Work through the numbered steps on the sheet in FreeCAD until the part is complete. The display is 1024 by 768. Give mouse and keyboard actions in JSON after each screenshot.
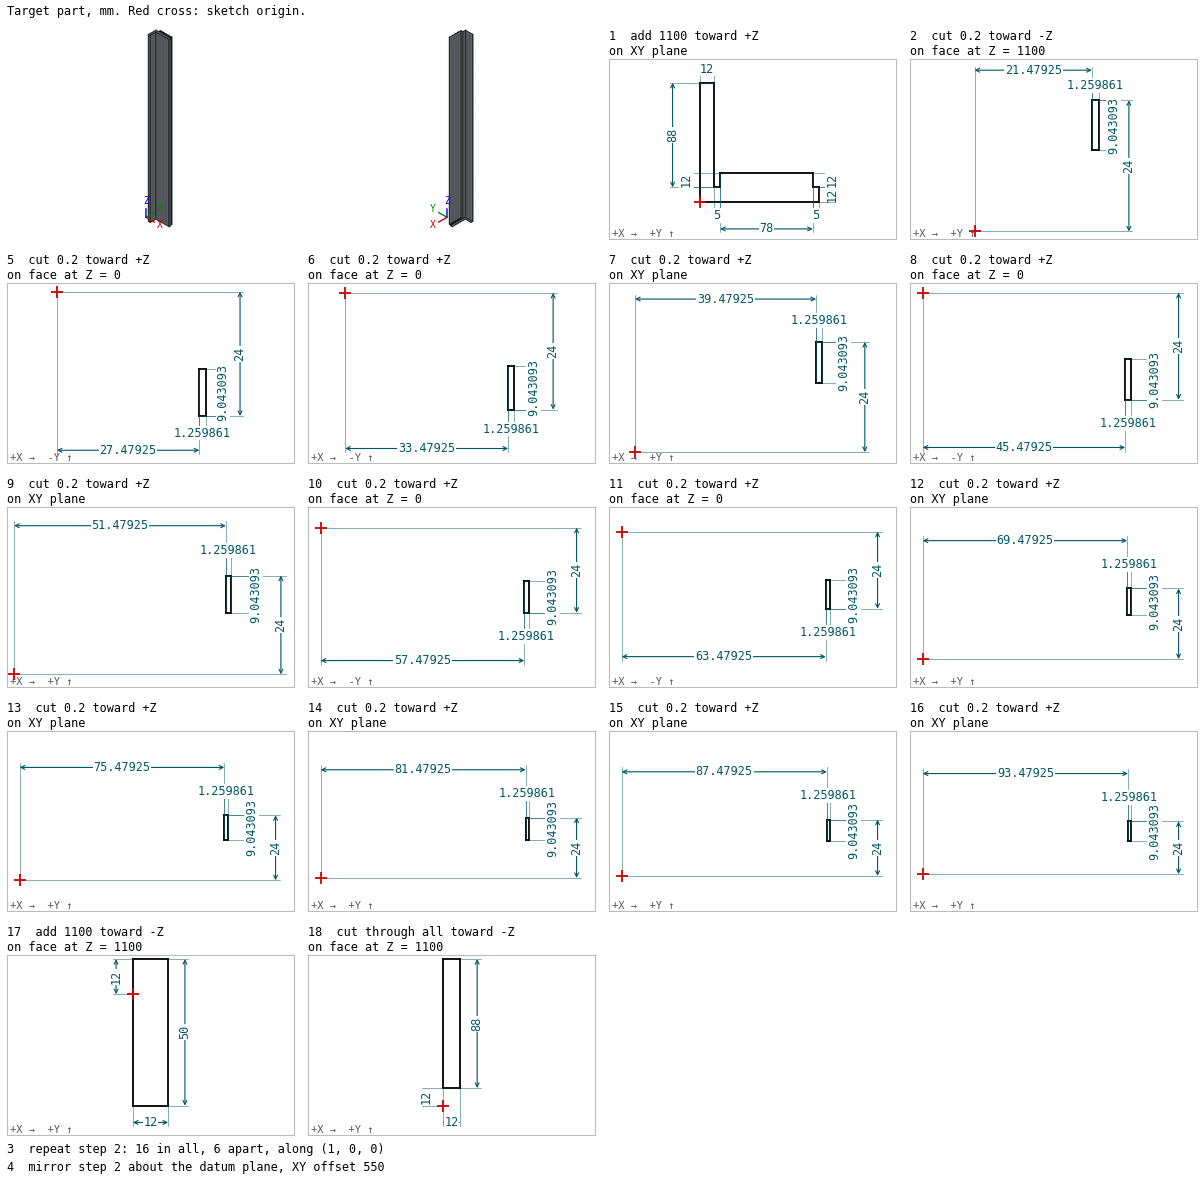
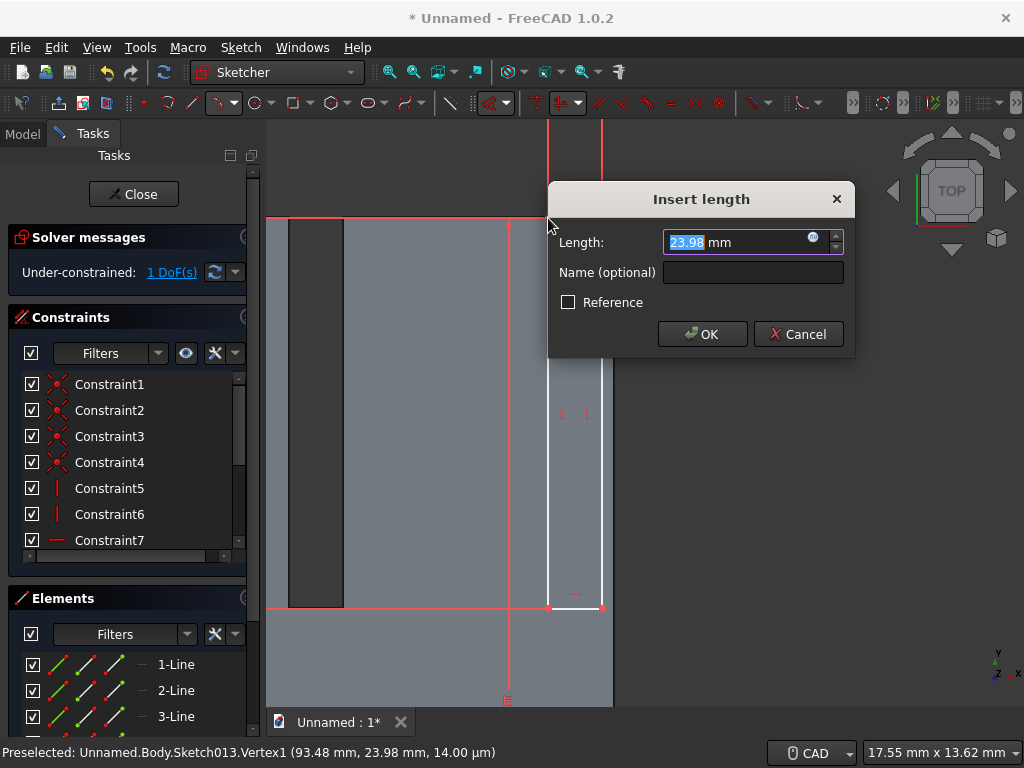
{"action": "type", "text": "24"}
{"action": "key", "text": "Return"}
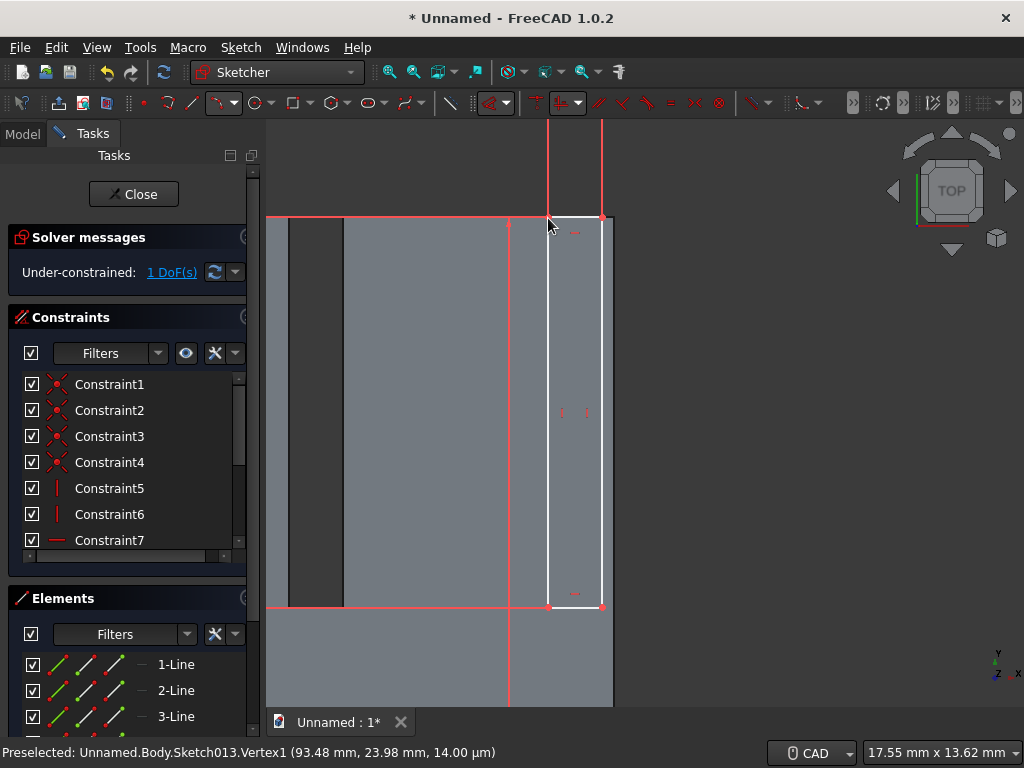
{"action": "left_click", "coordinate": [548, 217]}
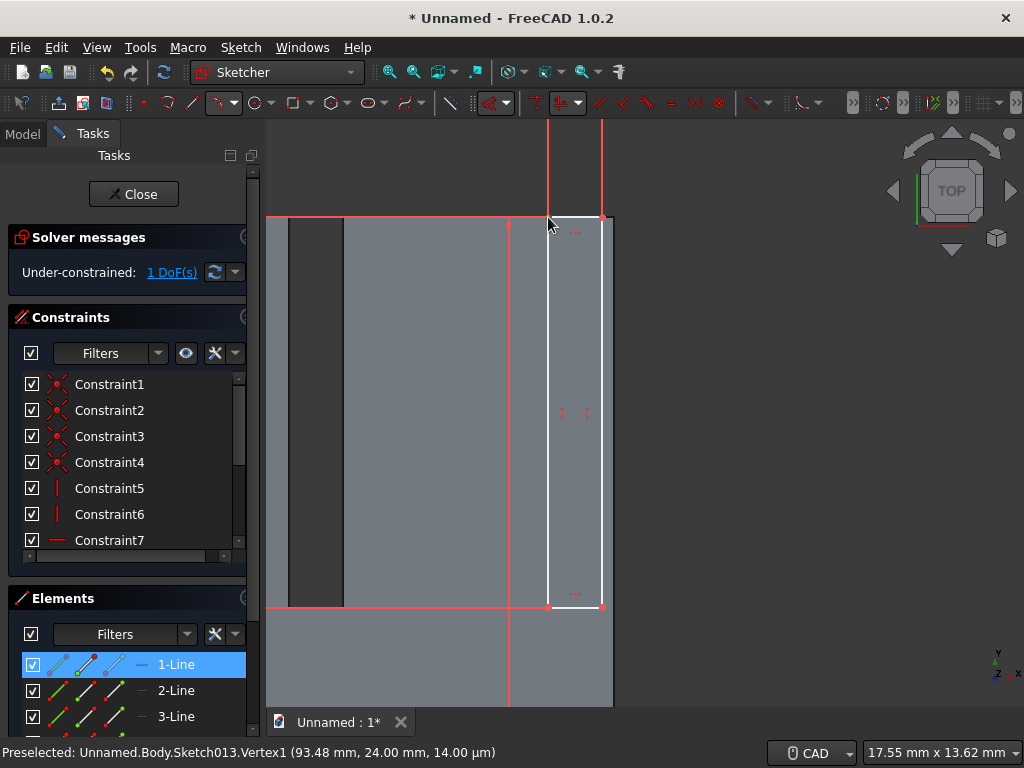
{"action": "key", "text": "l"}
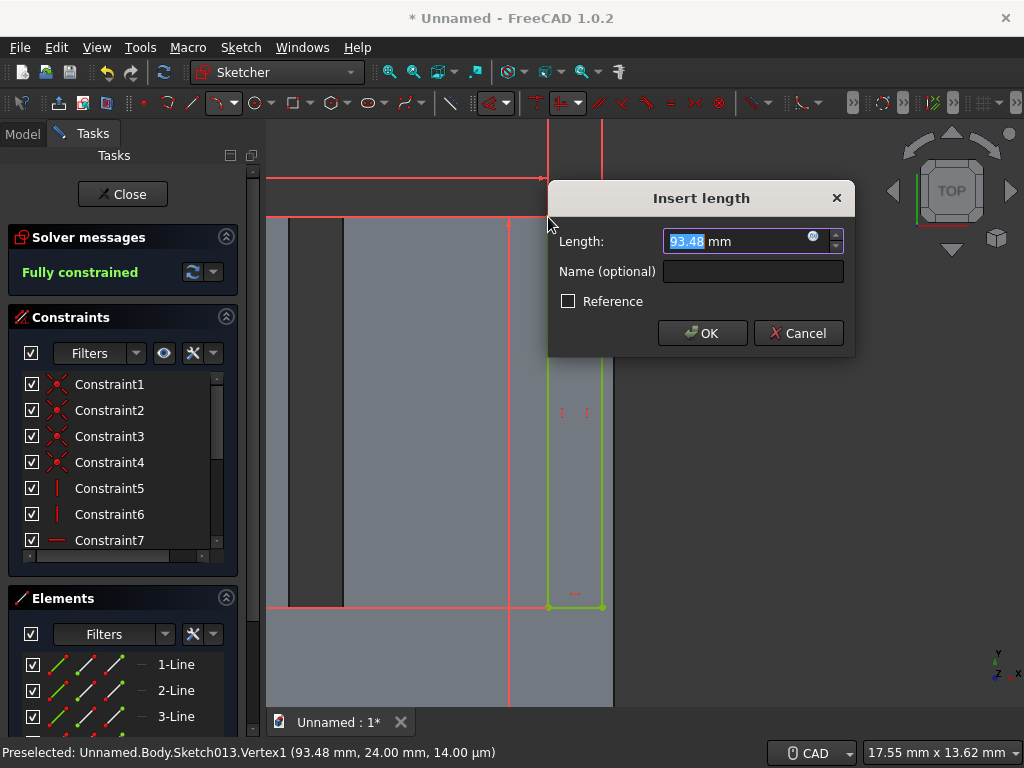
{"action": "type", "text": "93.47925"}
{"action": "key", "text": "Return"}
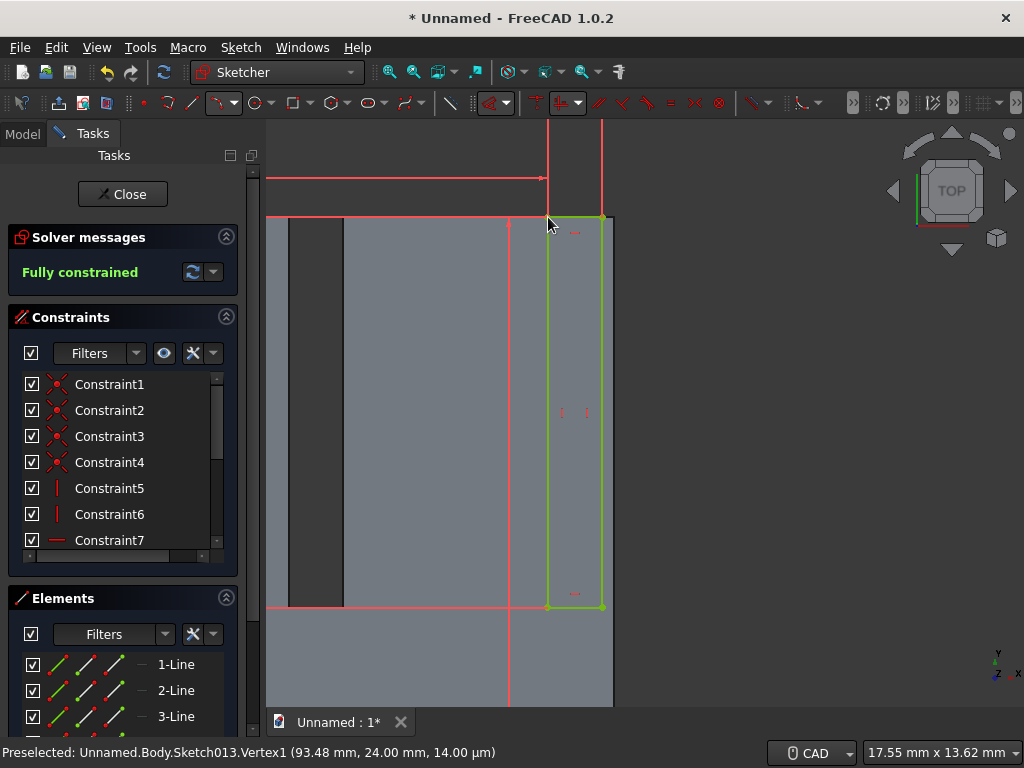
{"action": "left_click", "coordinate": [123, 194]}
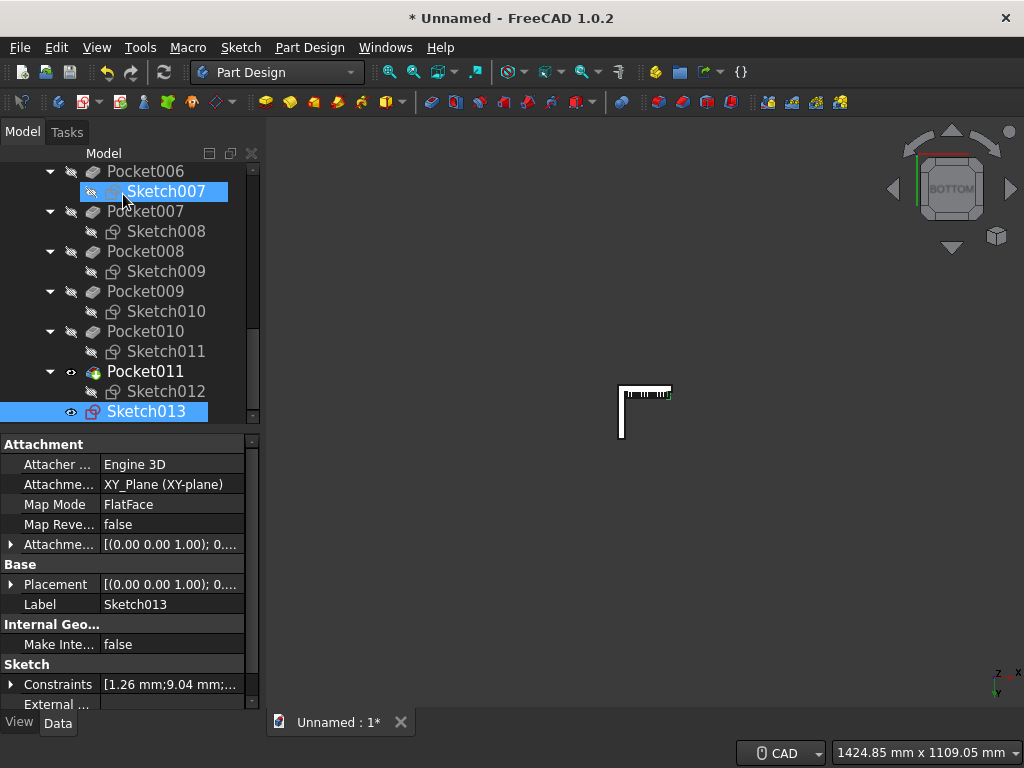
{"action": "left_click", "coordinate": [432, 102]}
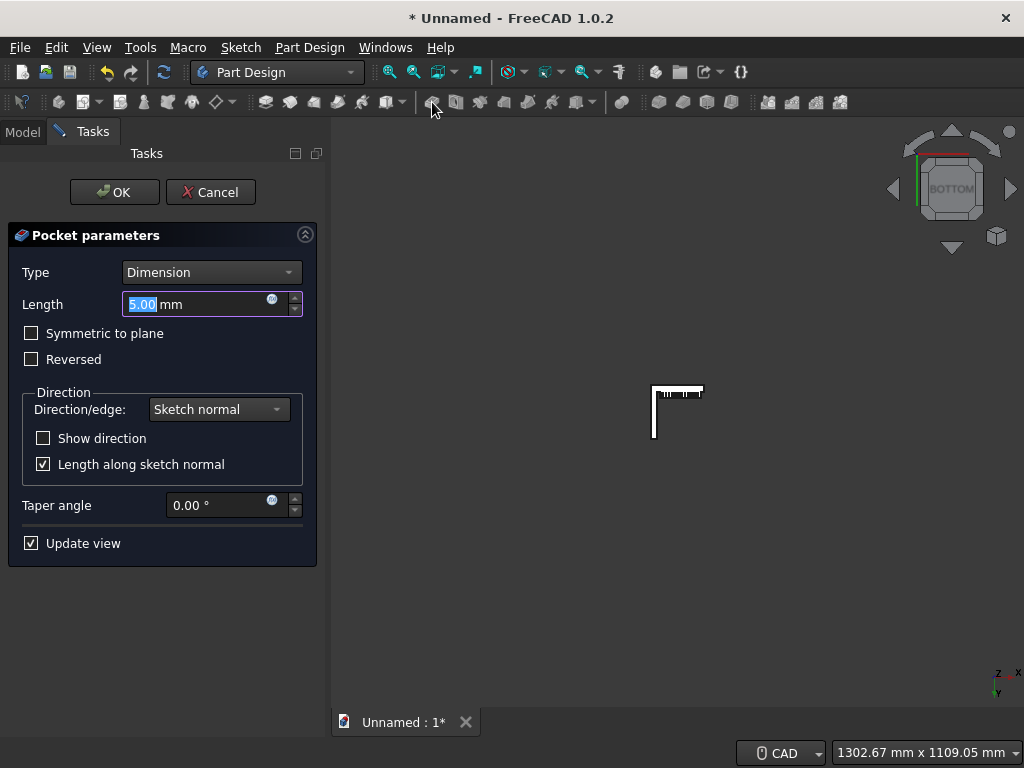
{"action": "type", "text": "0.2"}
{"action": "key", "text": "Tab"}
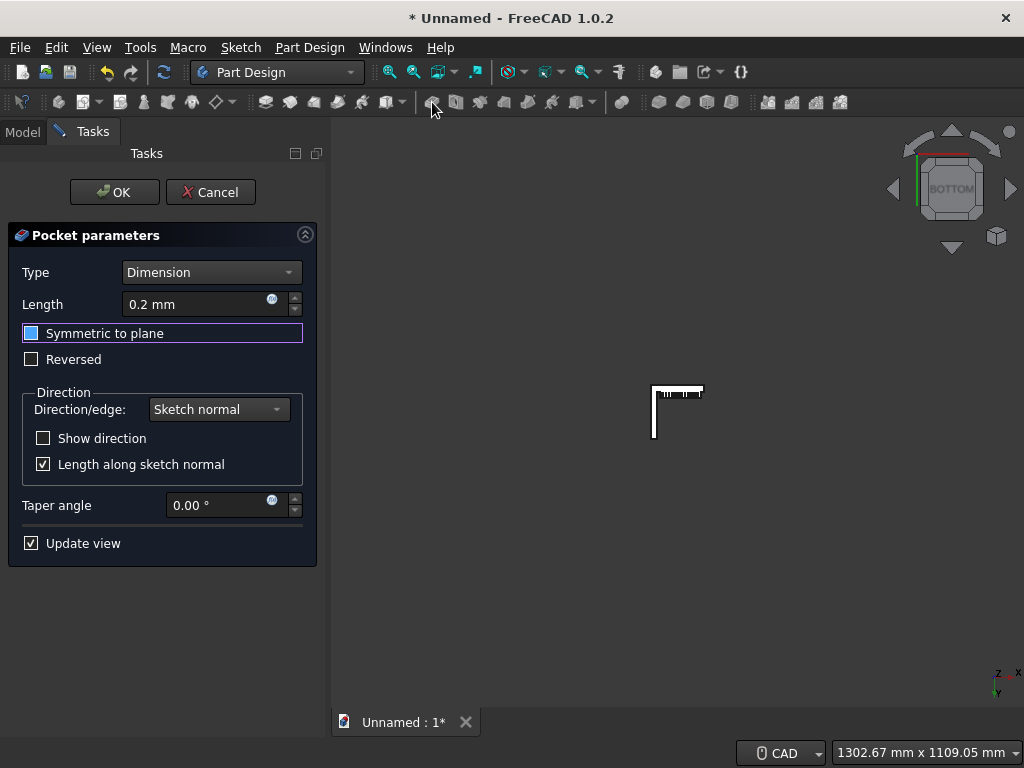
{"action": "left_click", "coordinate": [30, 359]}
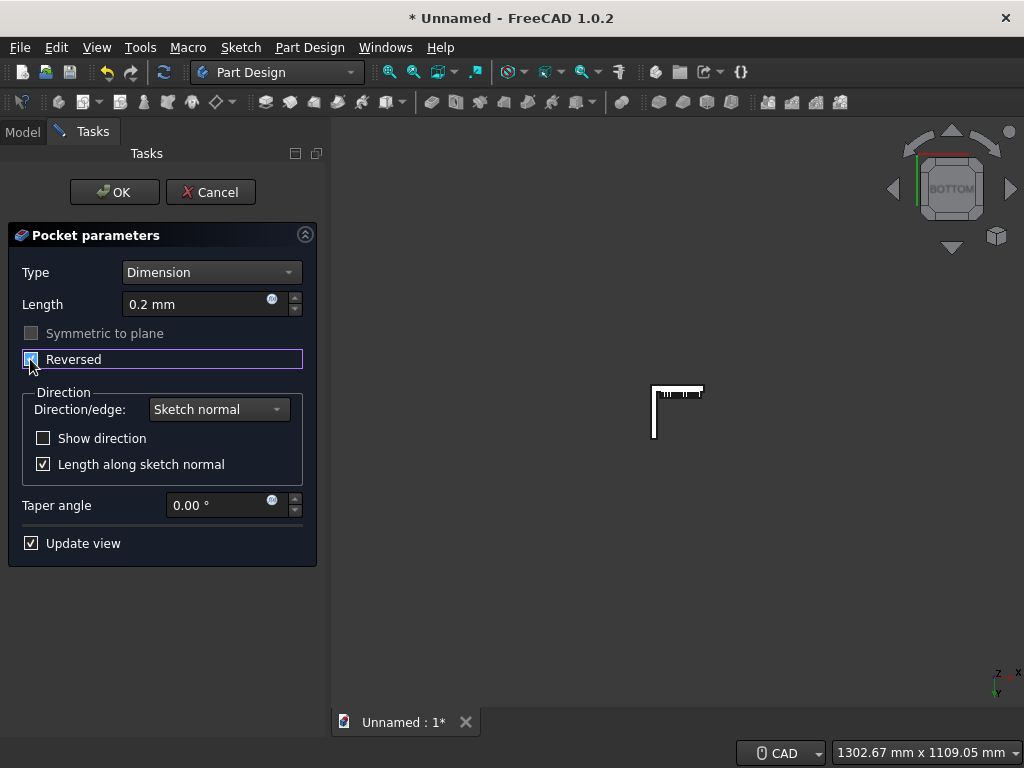
{"action": "left_click", "coordinate": [115, 192]}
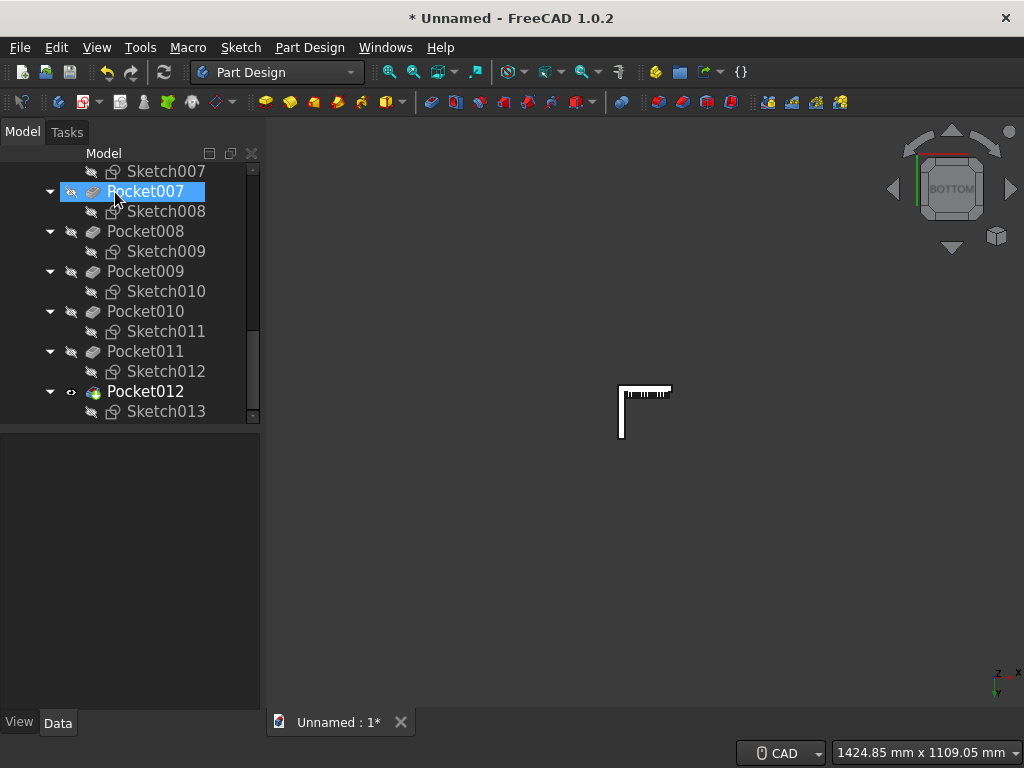
{"action": "left_click", "coordinate": [390, 72]}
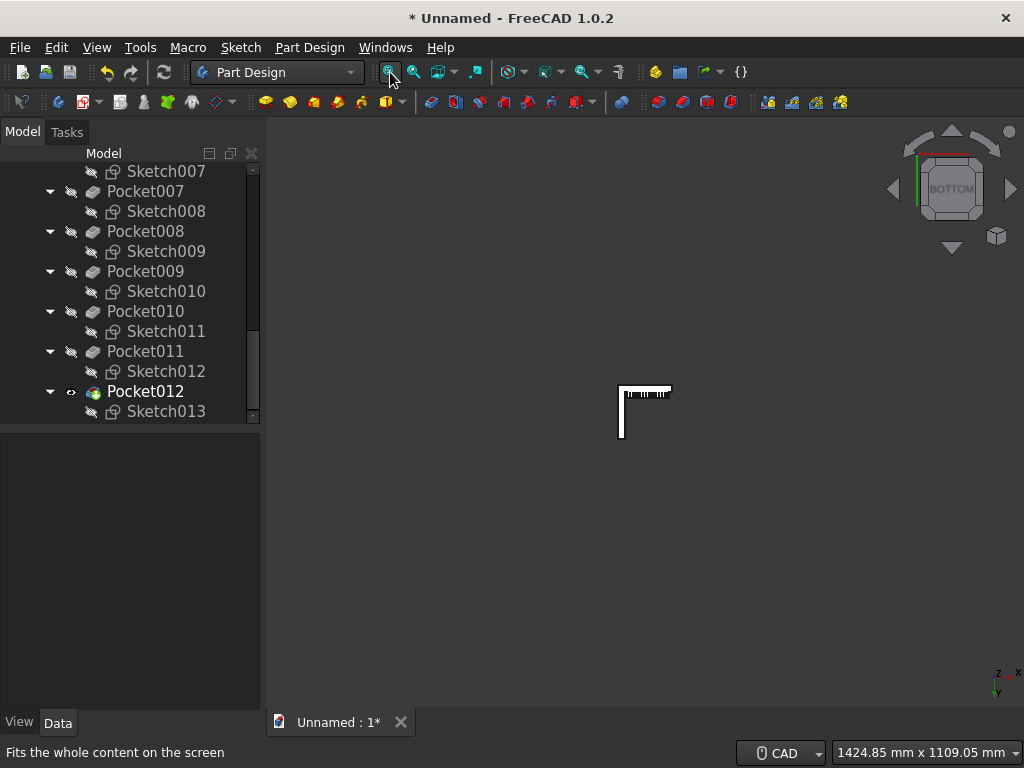
{"action": "key", "text": "0"}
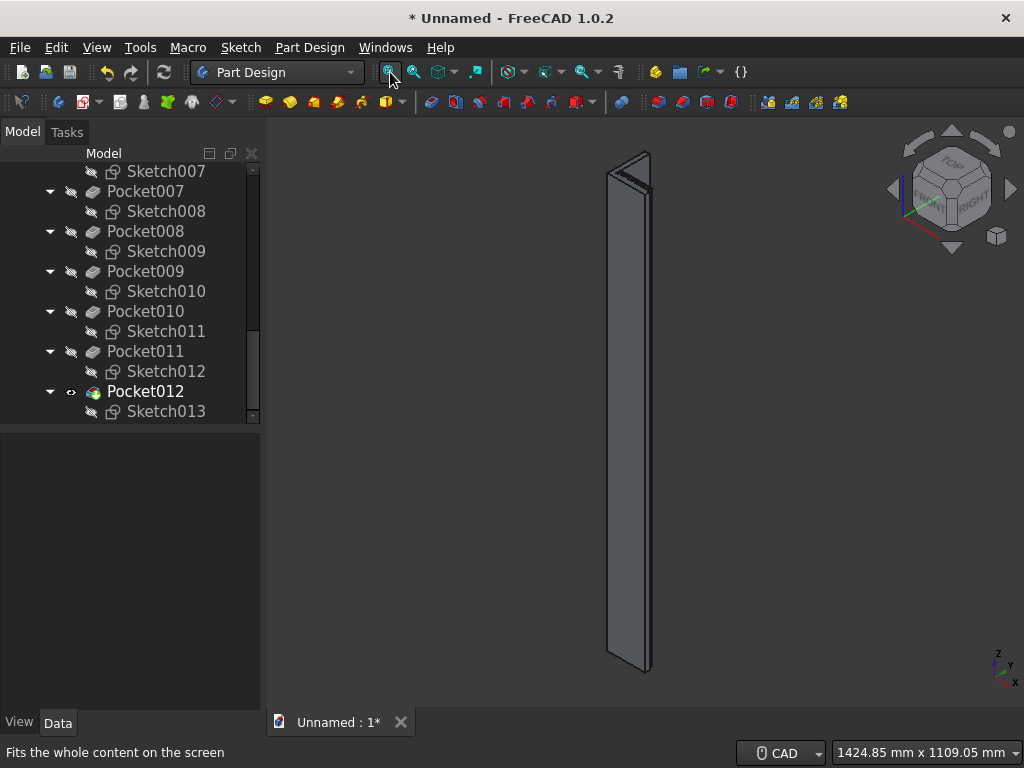
{"action": "scroll", "coordinate": [640, 188], "scroll_direction": "up", "scroll_amount": 6}